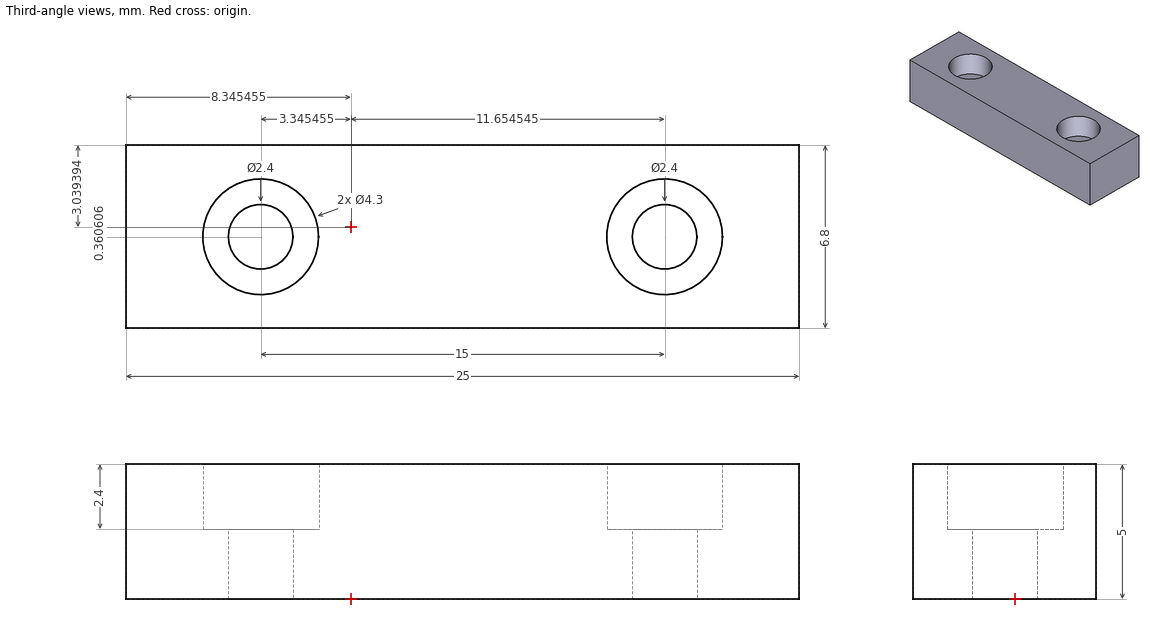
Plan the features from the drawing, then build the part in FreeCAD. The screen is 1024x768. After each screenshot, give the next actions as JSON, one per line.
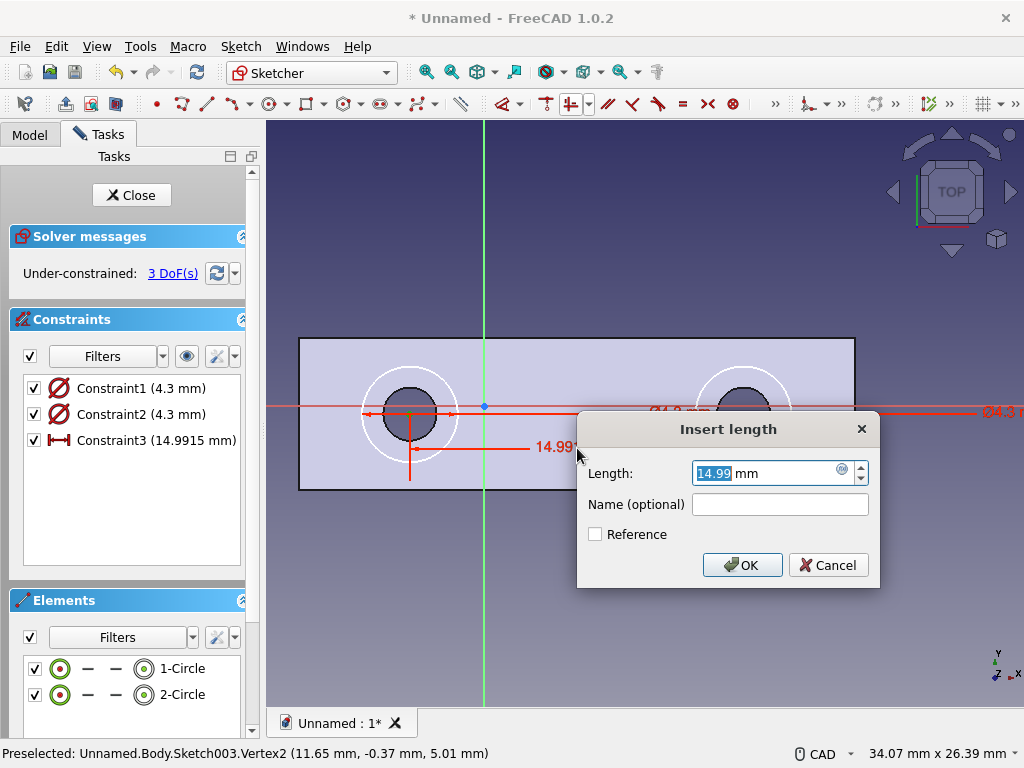
{"action": "type", "text": "15"}
{"action": "key", "text": "Return"}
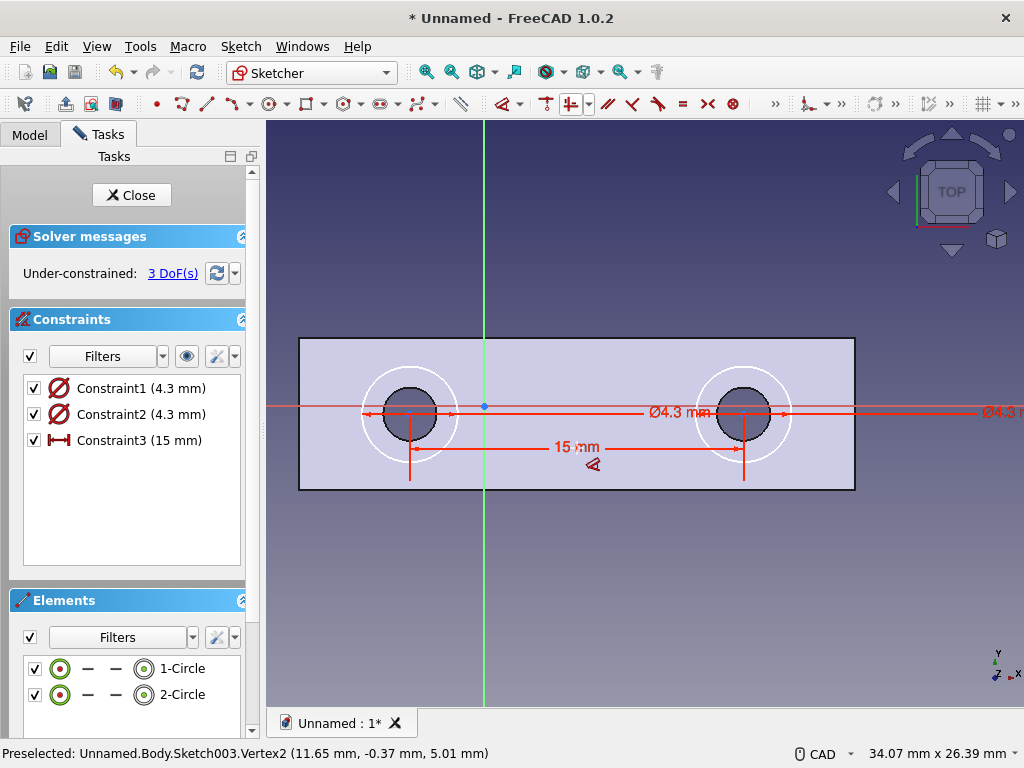
{"action": "left_click", "coordinate": [410, 414]}
{"action": "left_click", "coordinate": [464, 372]}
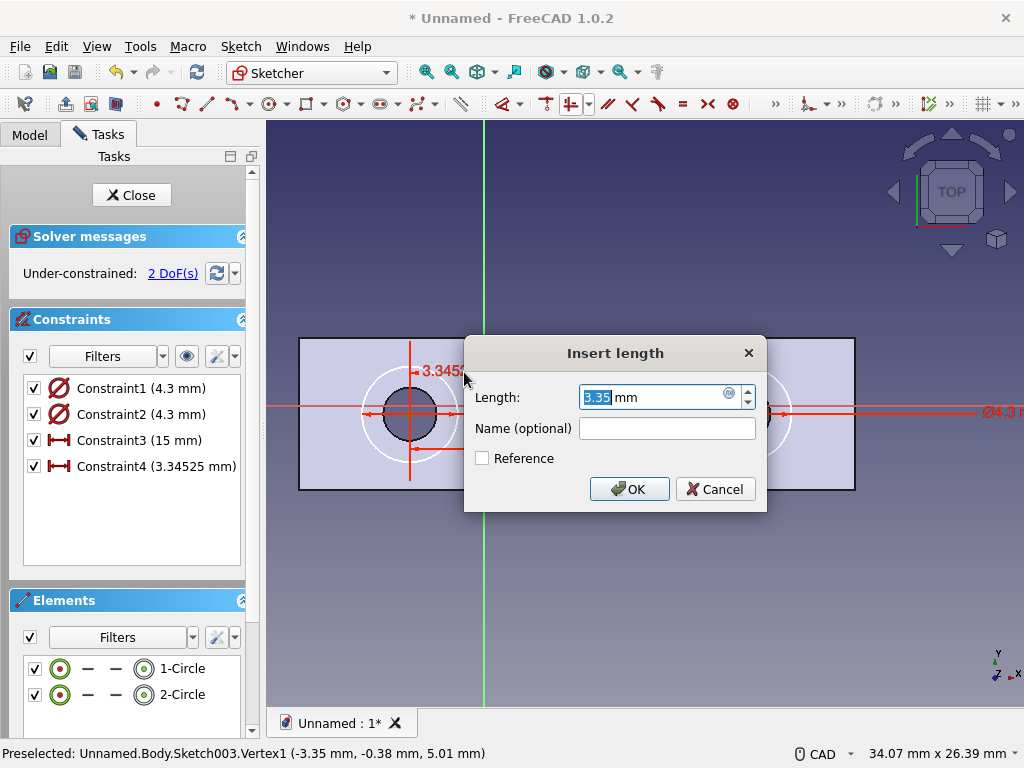
{"action": "type", "text": "3.345455"}
{"action": "key", "text": "Return"}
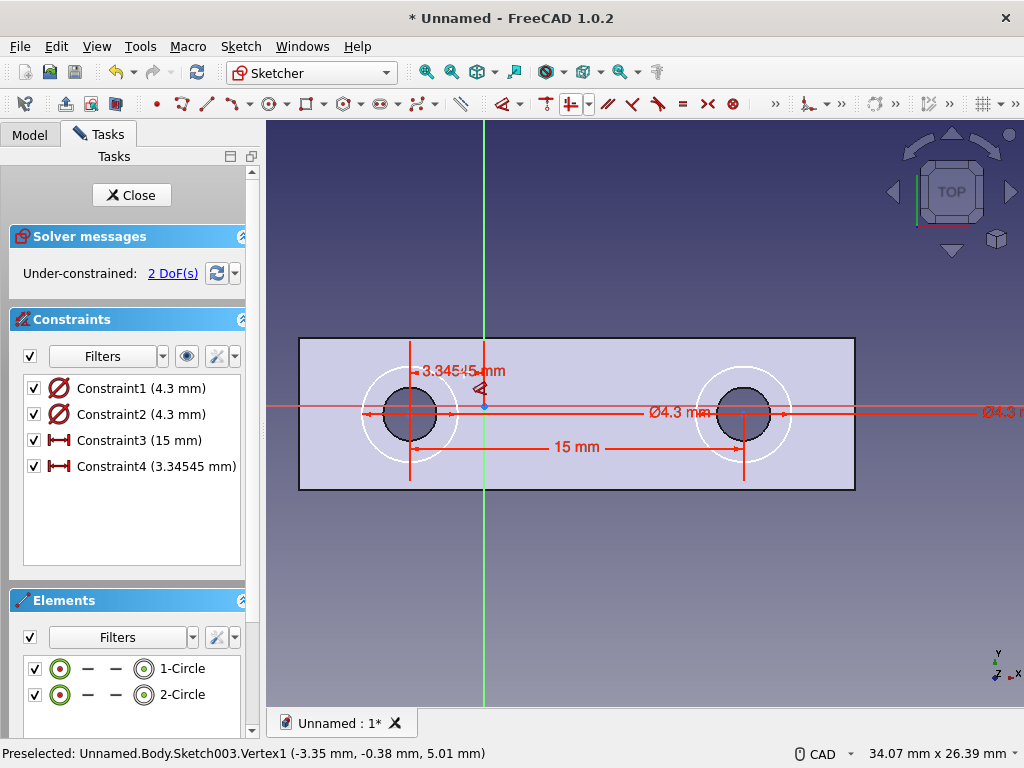
{"action": "scroll", "coordinate": [410, 414], "scroll_direction": "up", "scroll_amount": 8}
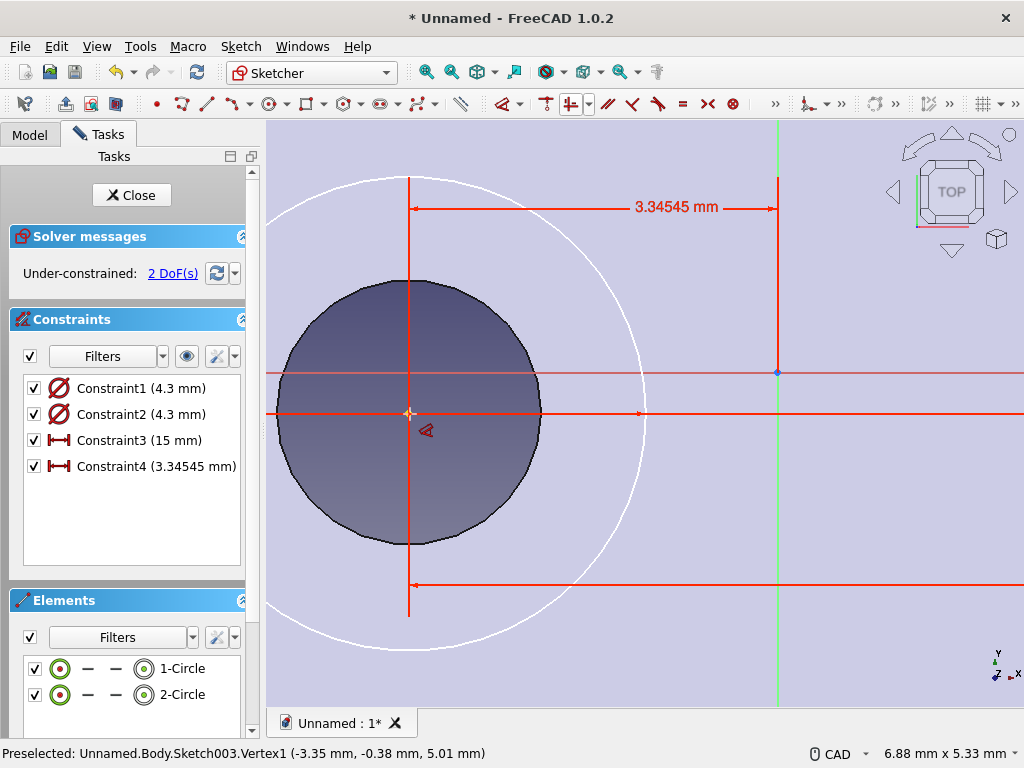
{"action": "left_click", "coordinate": [409, 414]}
{"action": "left_click", "coordinate": [375, 393]}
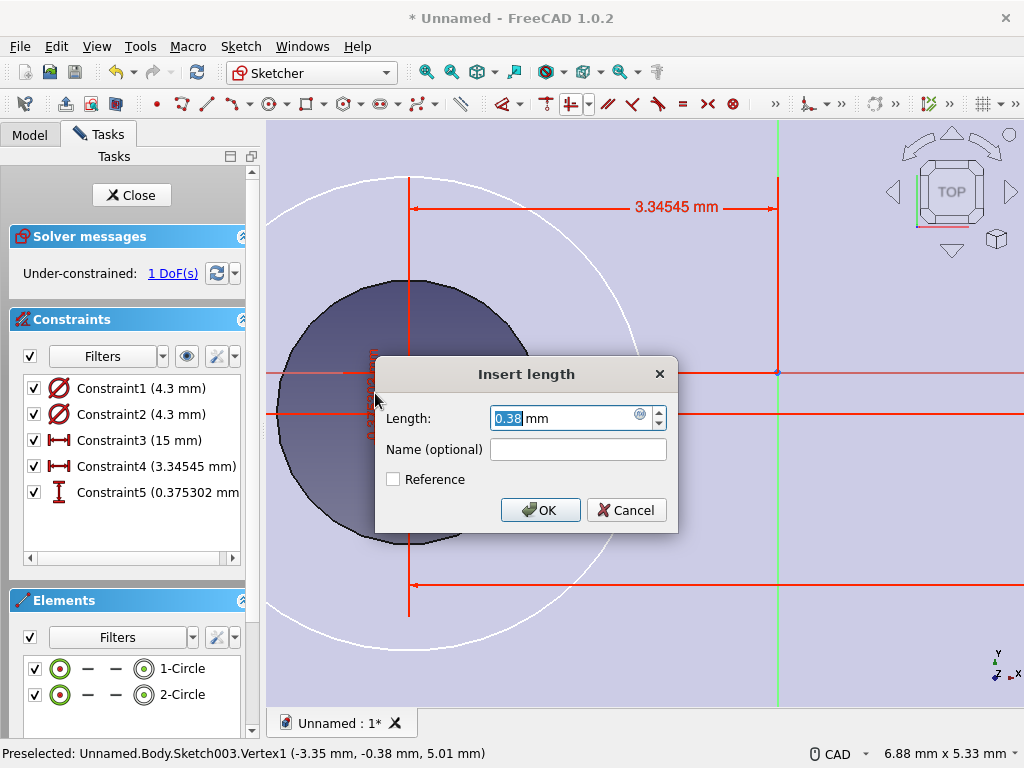
{"action": "type", "text": "0.360606"}
{"action": "key", "text": "Return"}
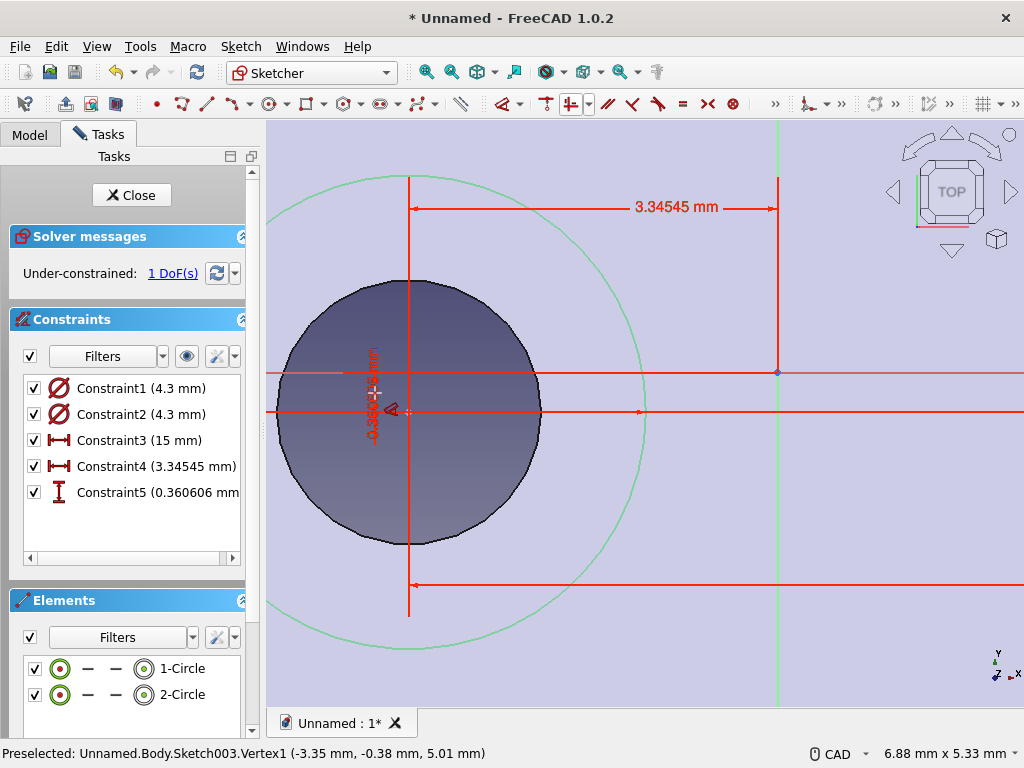
{"action": "scroll", "coordinate": [410, 414], "scroll_direction": "down", "scroll_amount": 8}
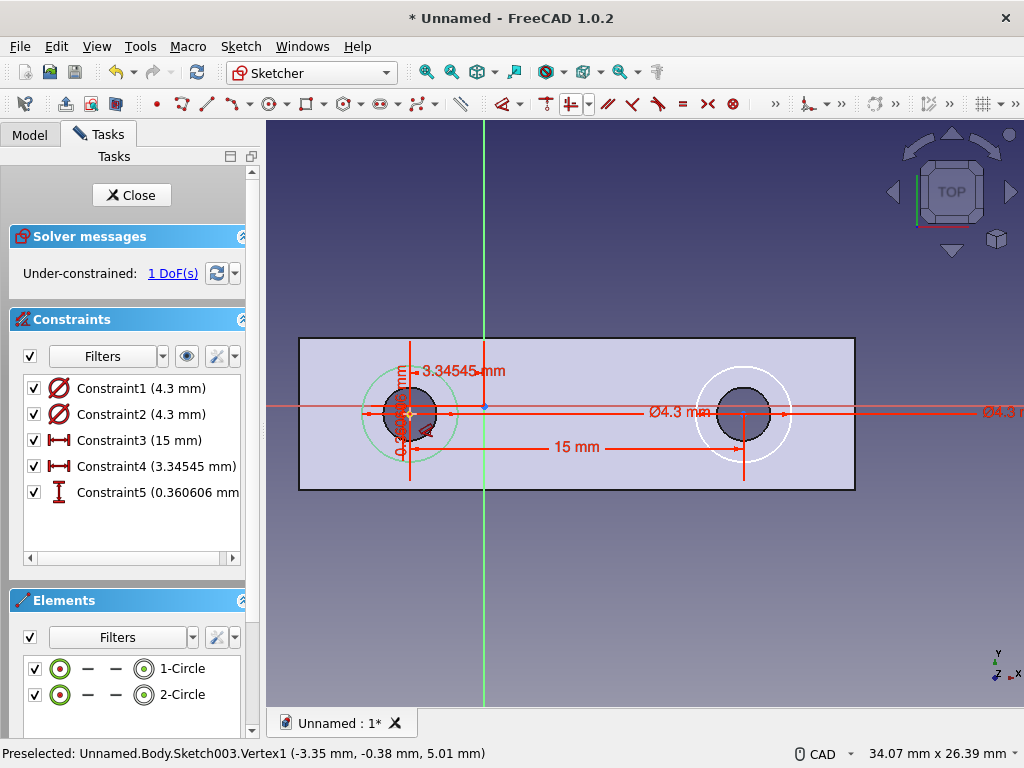
{"action": "scroll", "coordinate": [744, 414], "scroll_direction": "up", "scroll_amount": 8}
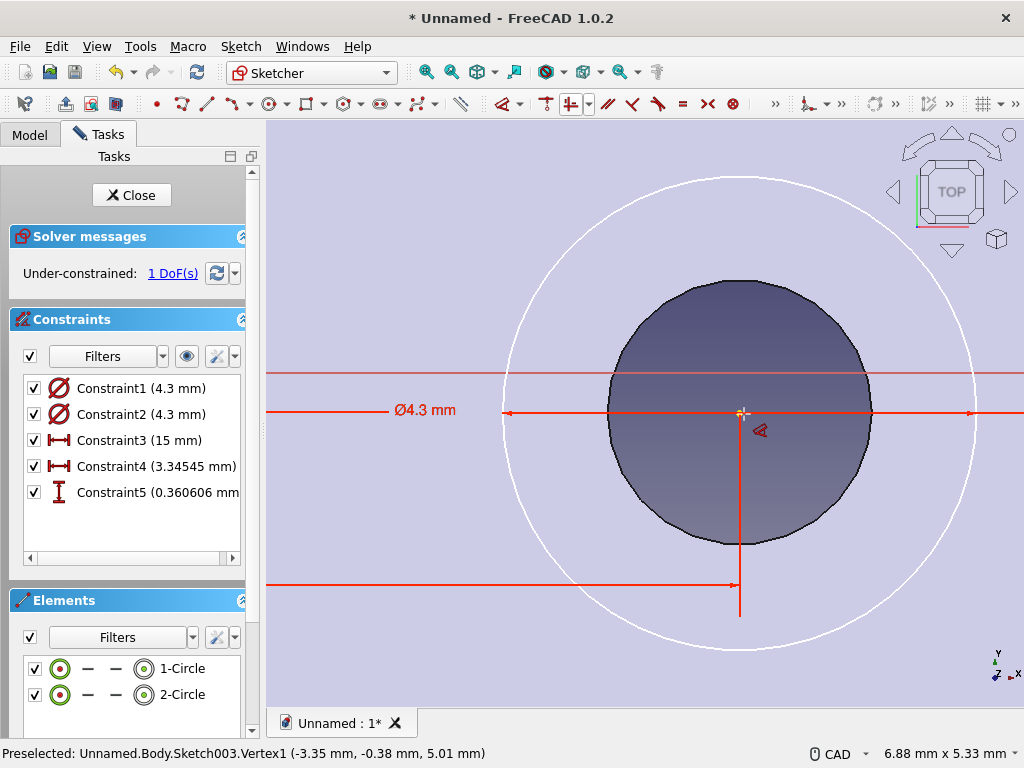
{"action": "left_click", "coordinate": [740, 413]}
{"action": "left_click", "coordinate": [774, 393]}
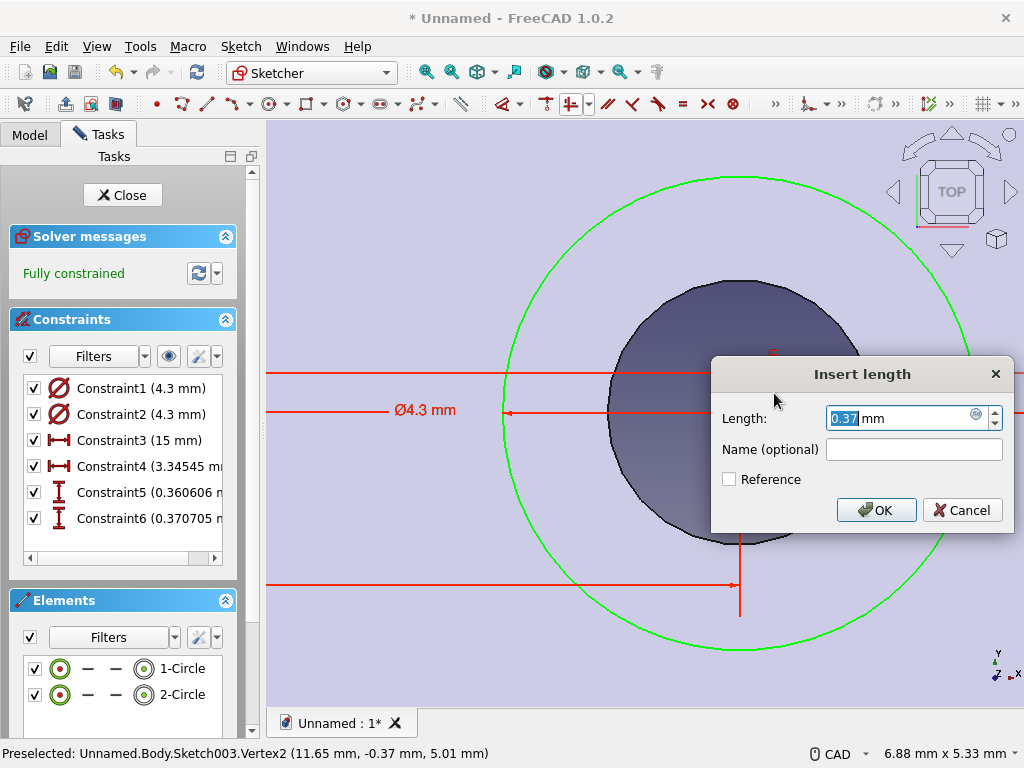
{"action": "type", "text": "0.360606"}
{"action": "key", "text": "Return"}
{"action": "key", "text": "Escape"}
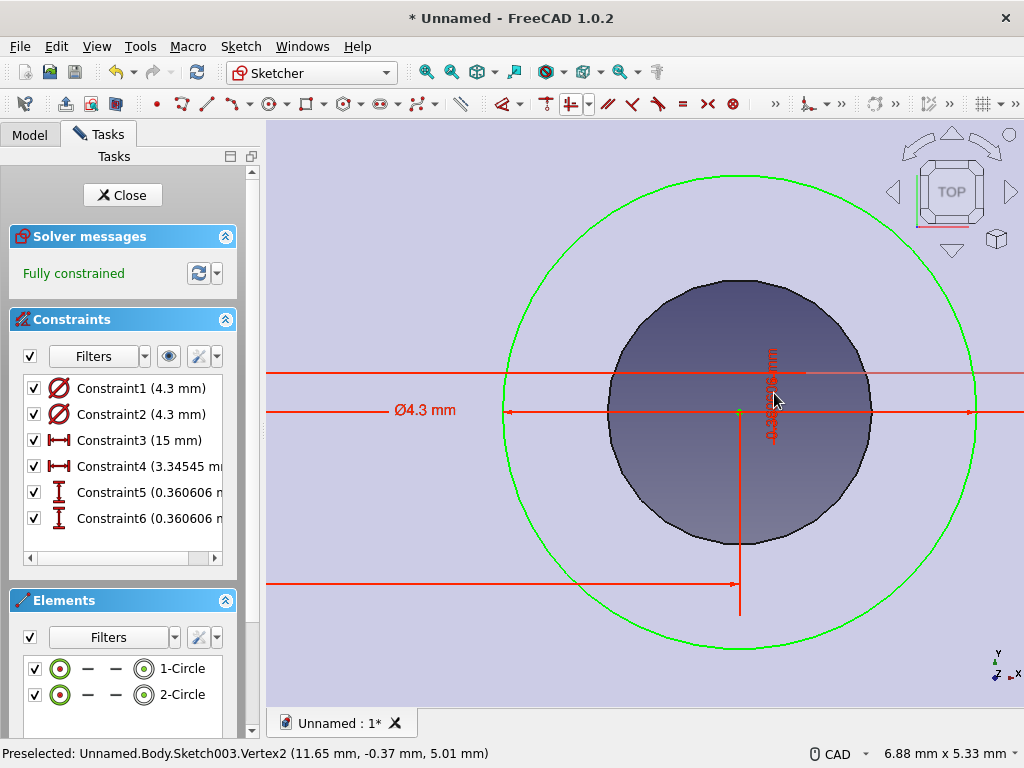
{"action": "left_click", "coordinate": [123, 195]}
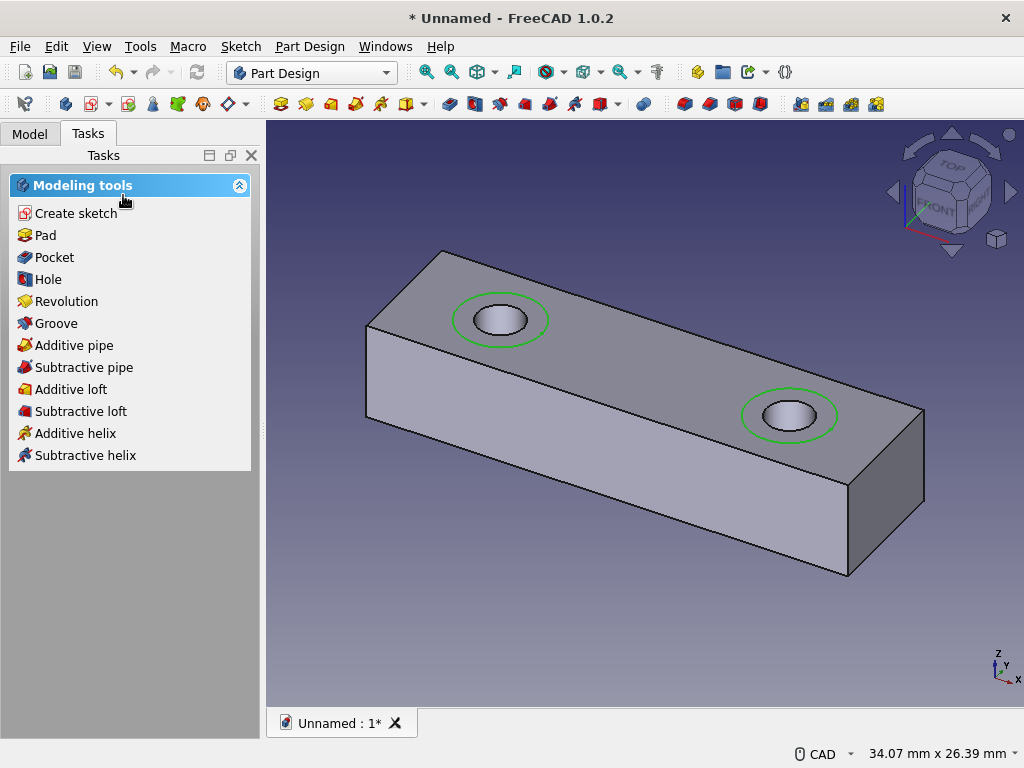
{"action": "left_click", "coordinate": [450, 104]}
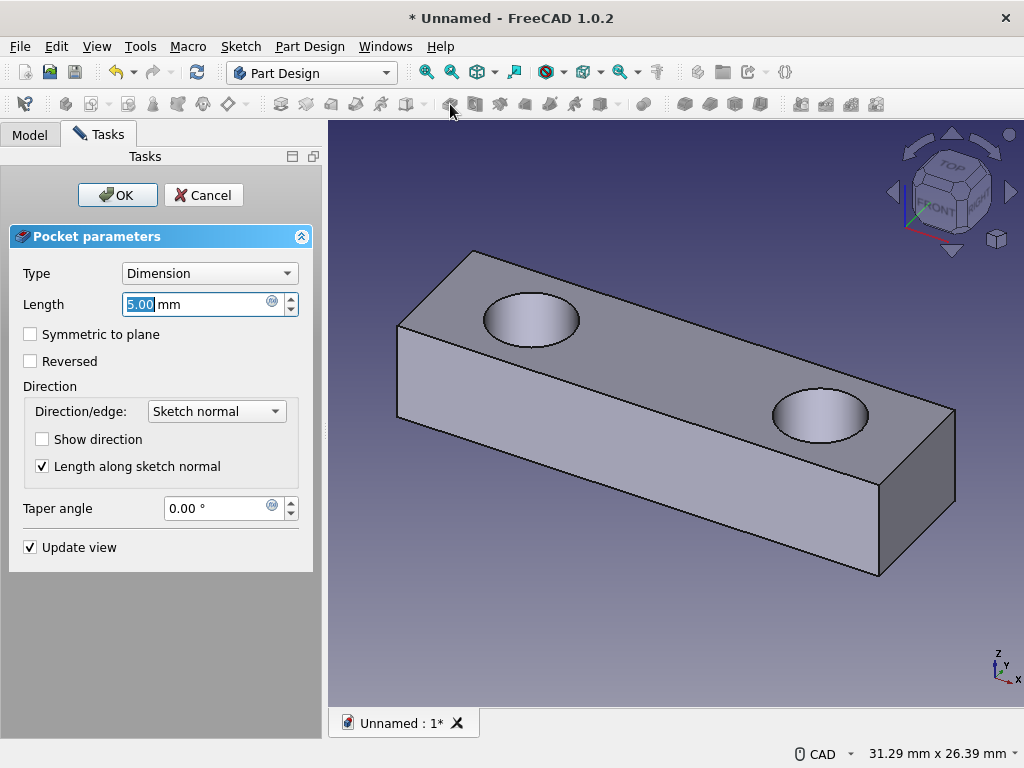
{"action": "type", "text": "2.4"}
{"action": "key", "text": "Tab"}